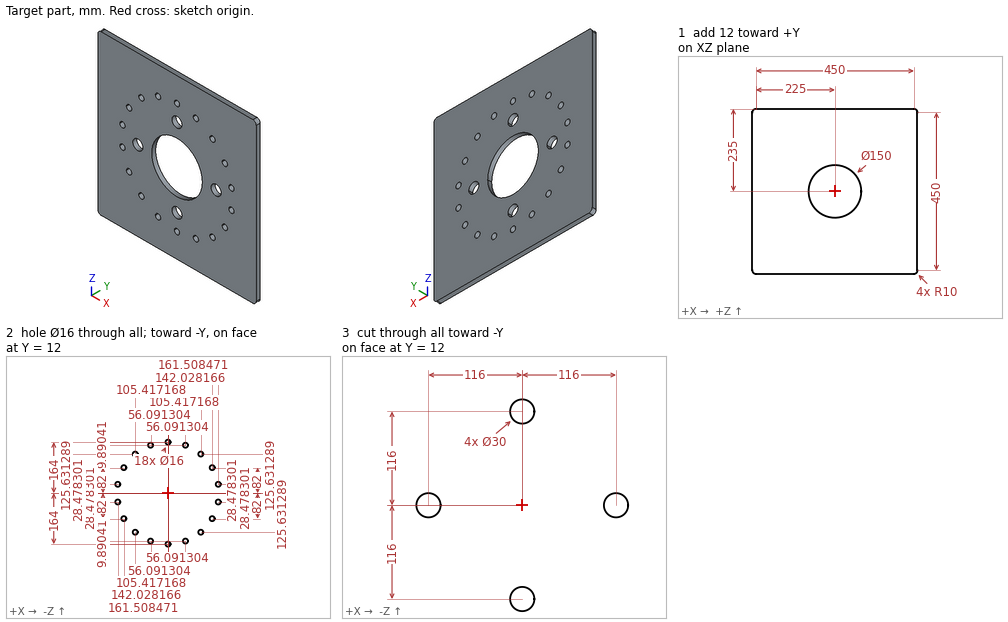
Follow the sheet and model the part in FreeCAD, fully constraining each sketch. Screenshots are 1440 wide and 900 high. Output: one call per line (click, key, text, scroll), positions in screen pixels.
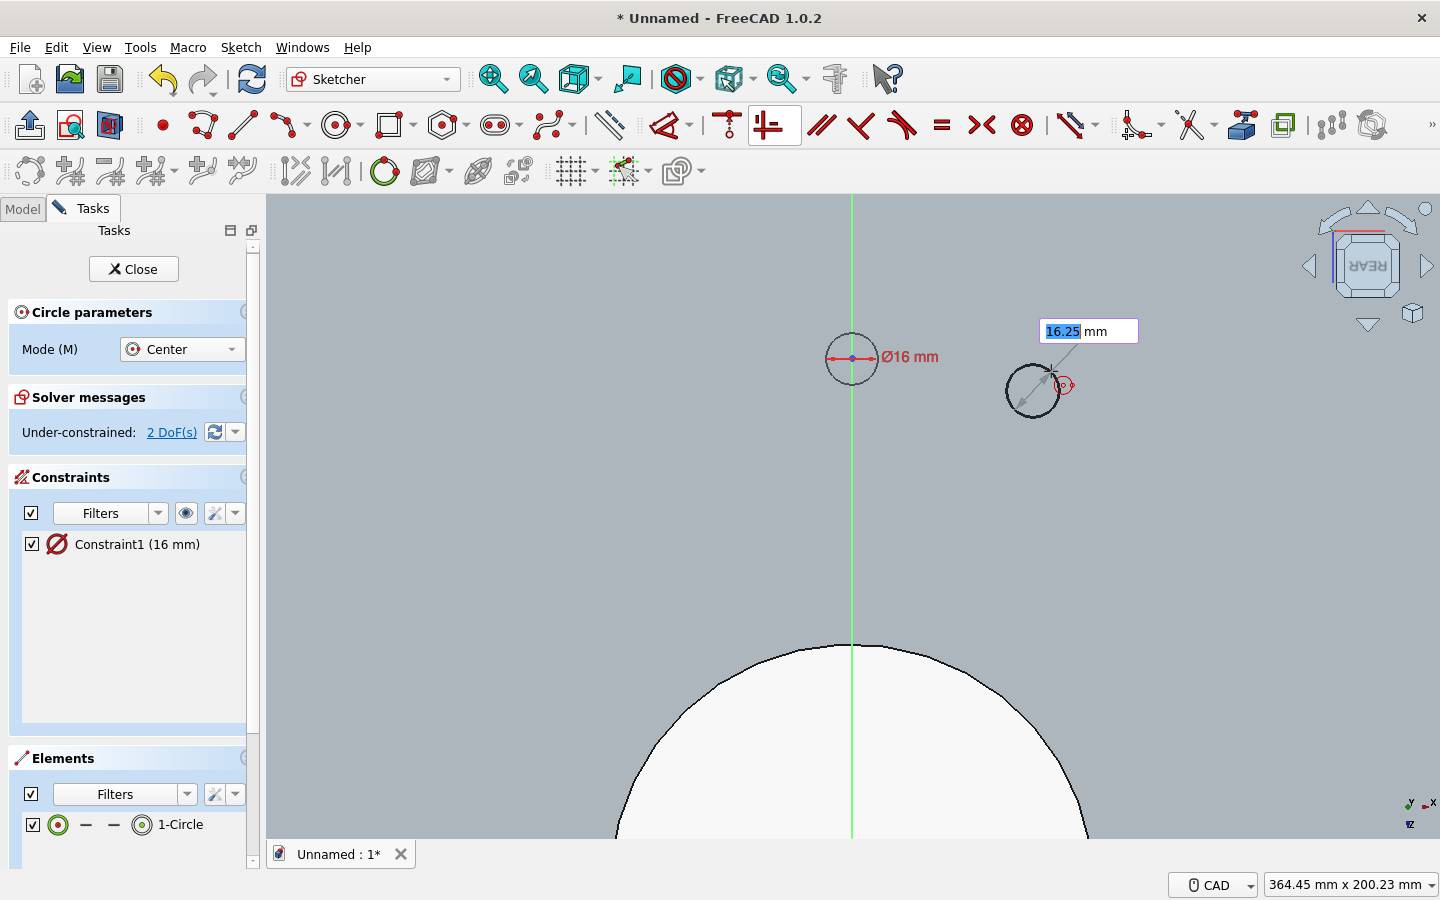
text(16)
key(Return)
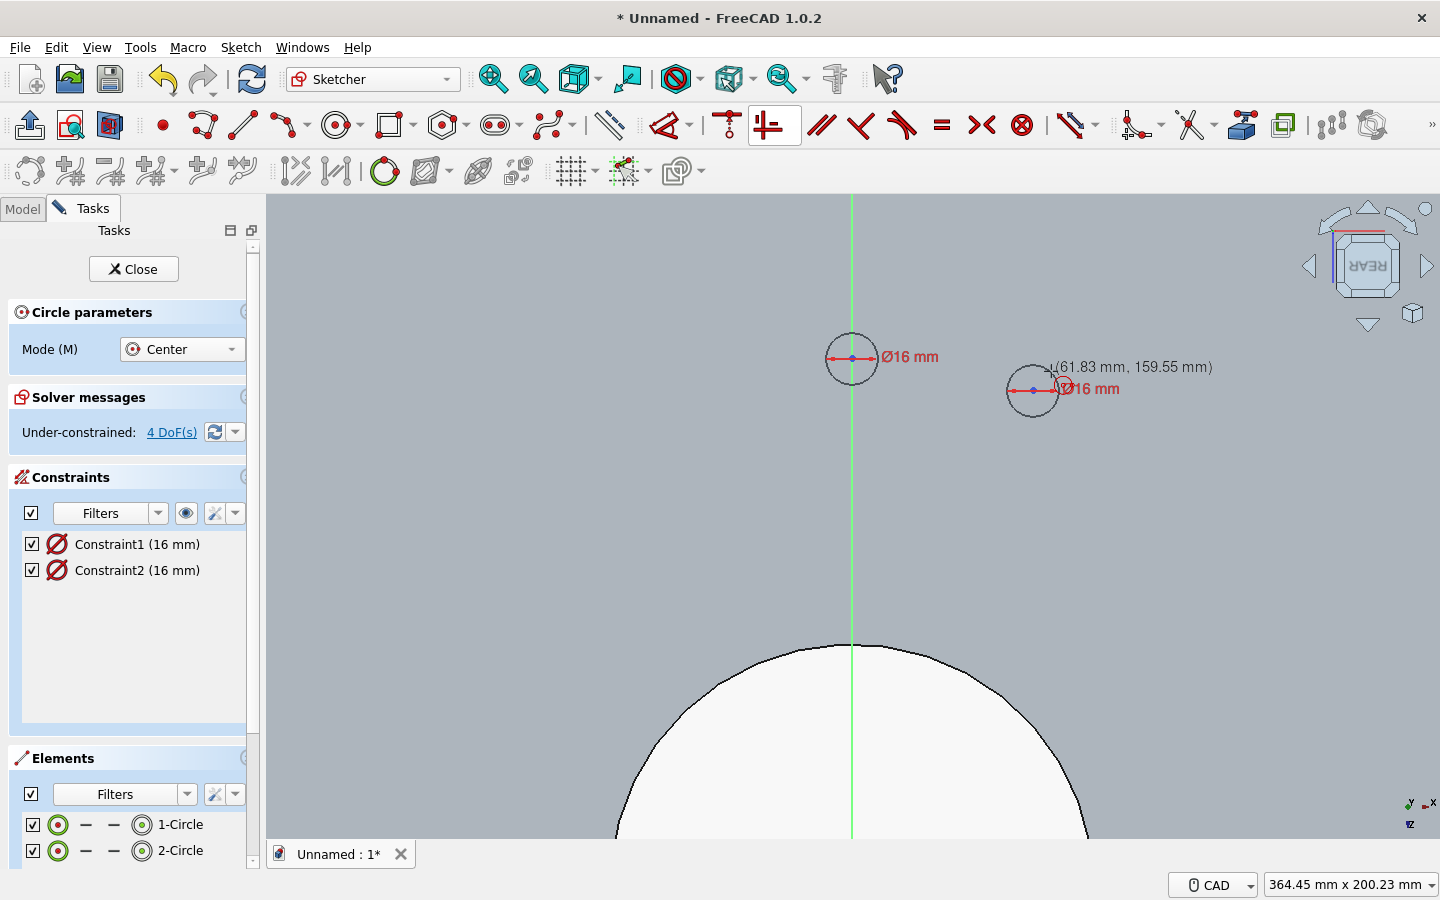
click(1191, 481)
move(1210, 463)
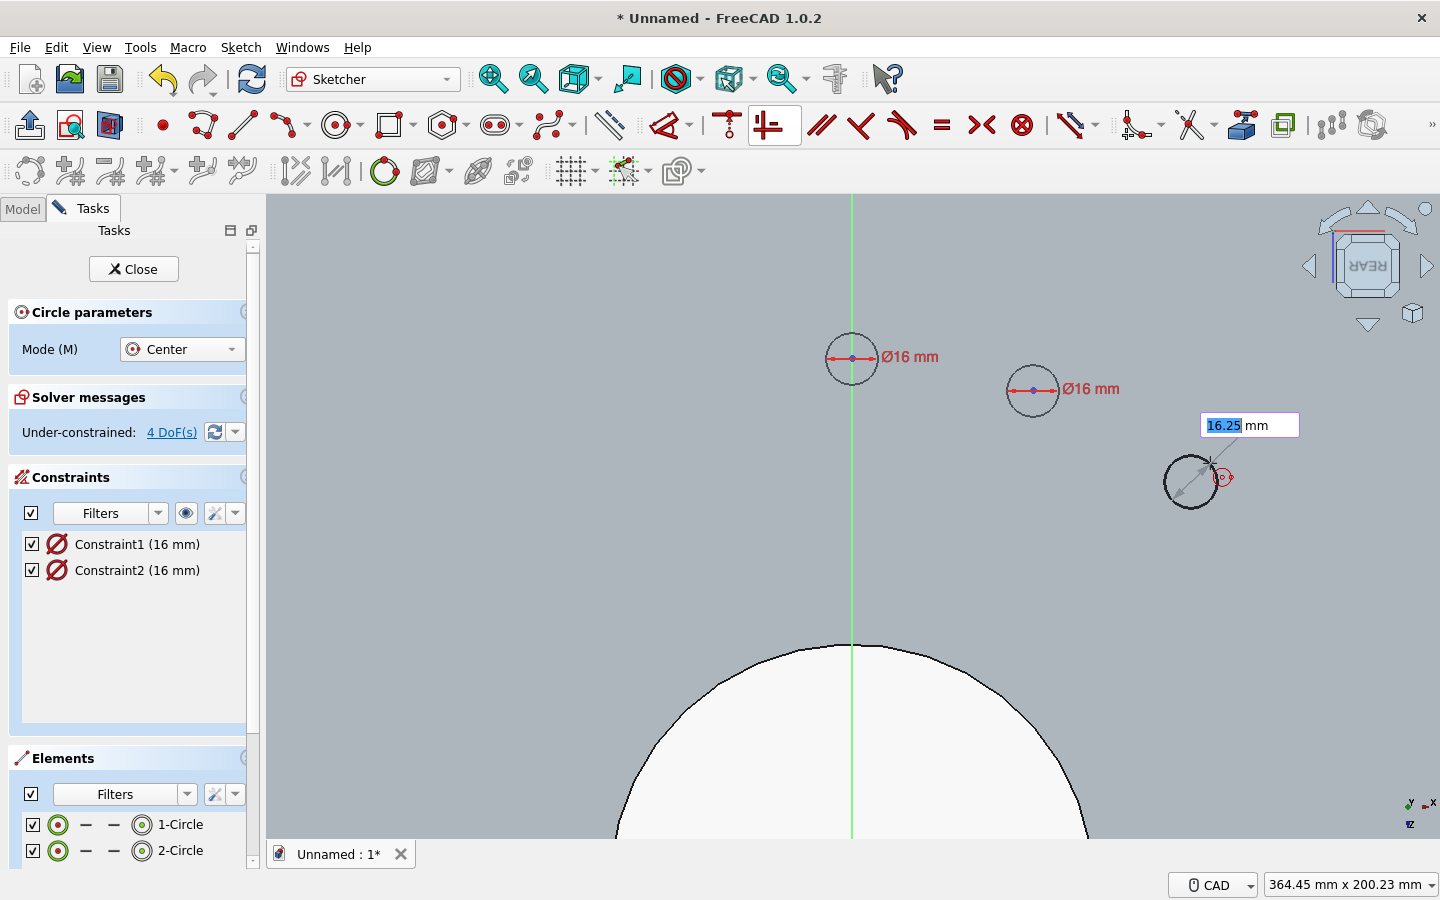
text(16)
key(Return)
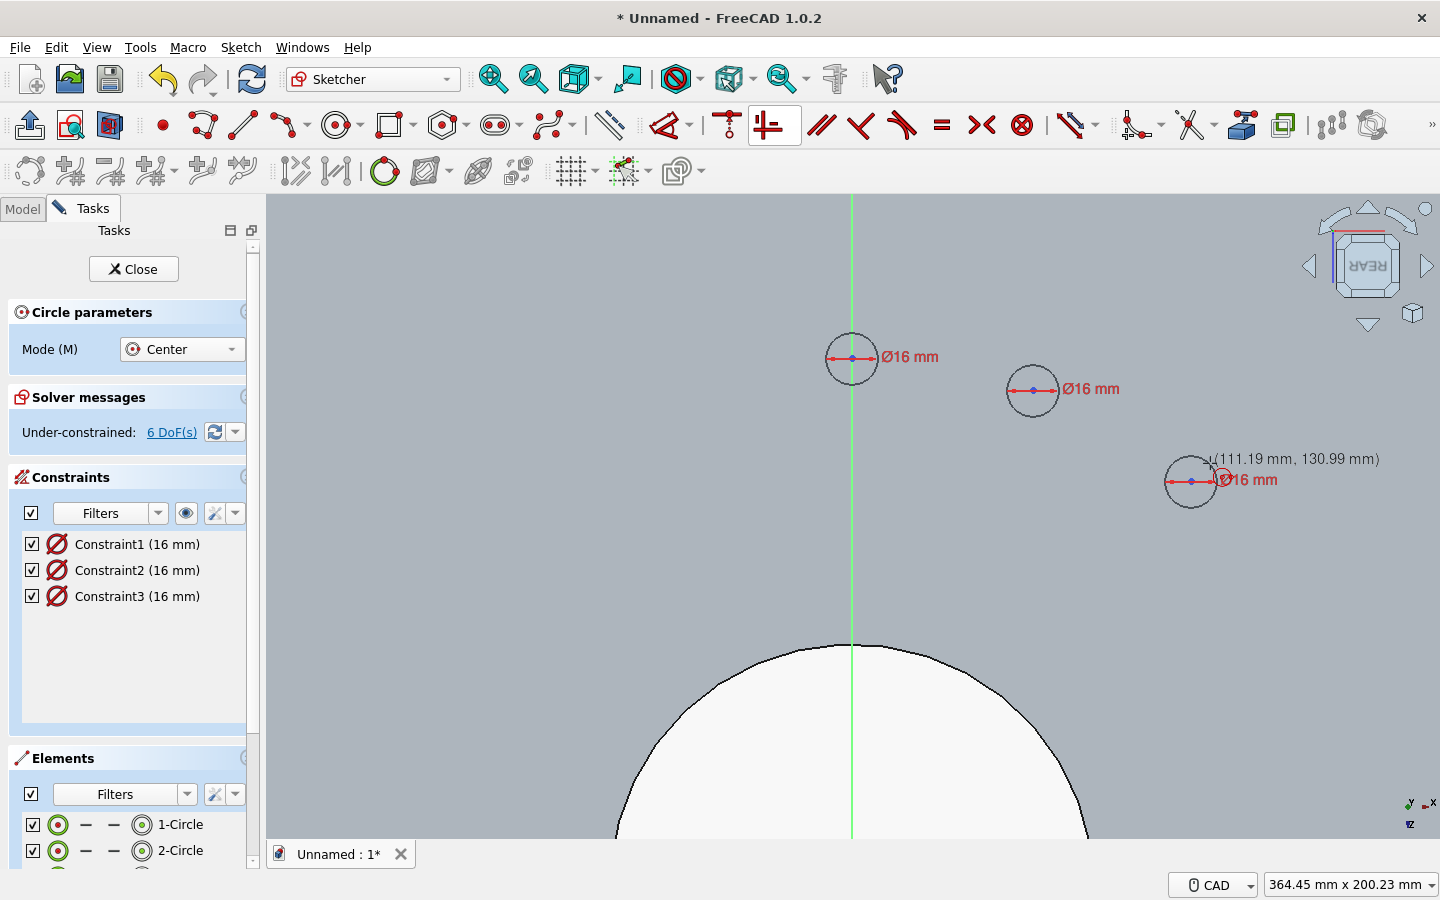
scroll(745, 301, down, 5)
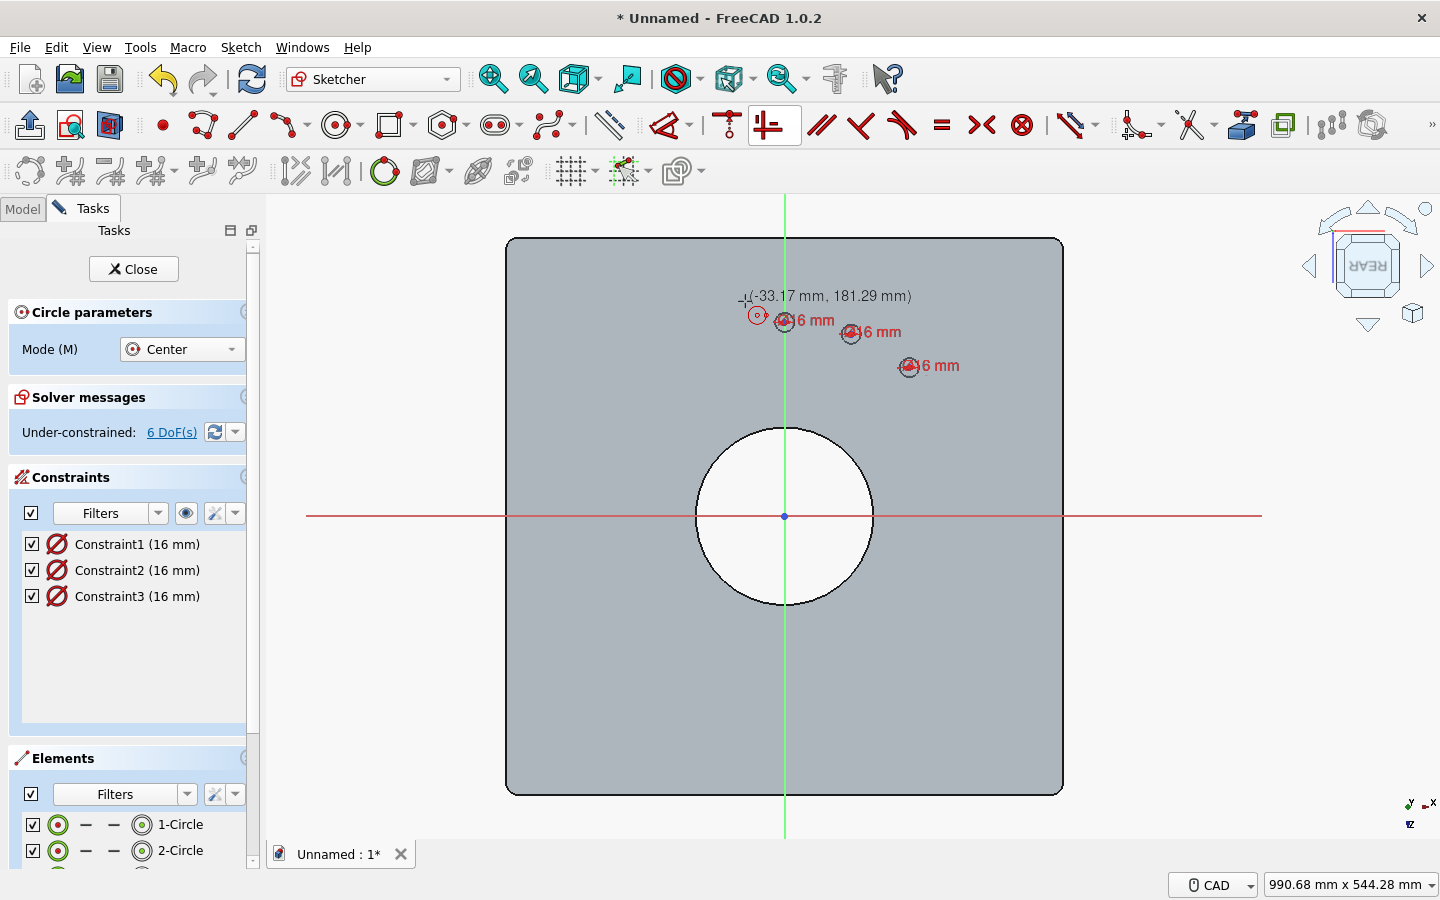
scroll(953, 419, up, 5)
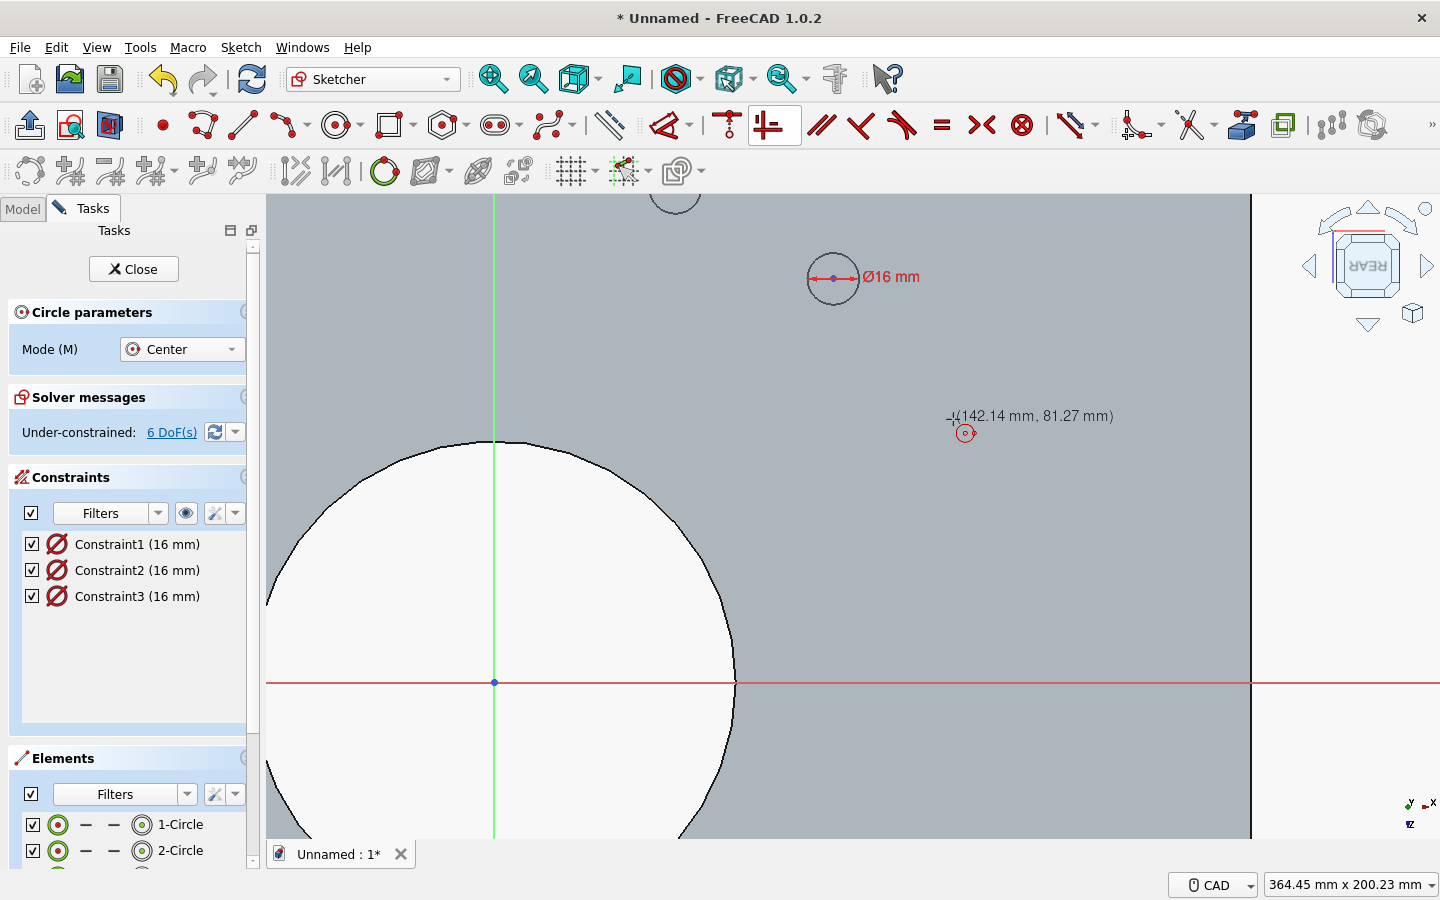
click(952, 419)
move(970, 401)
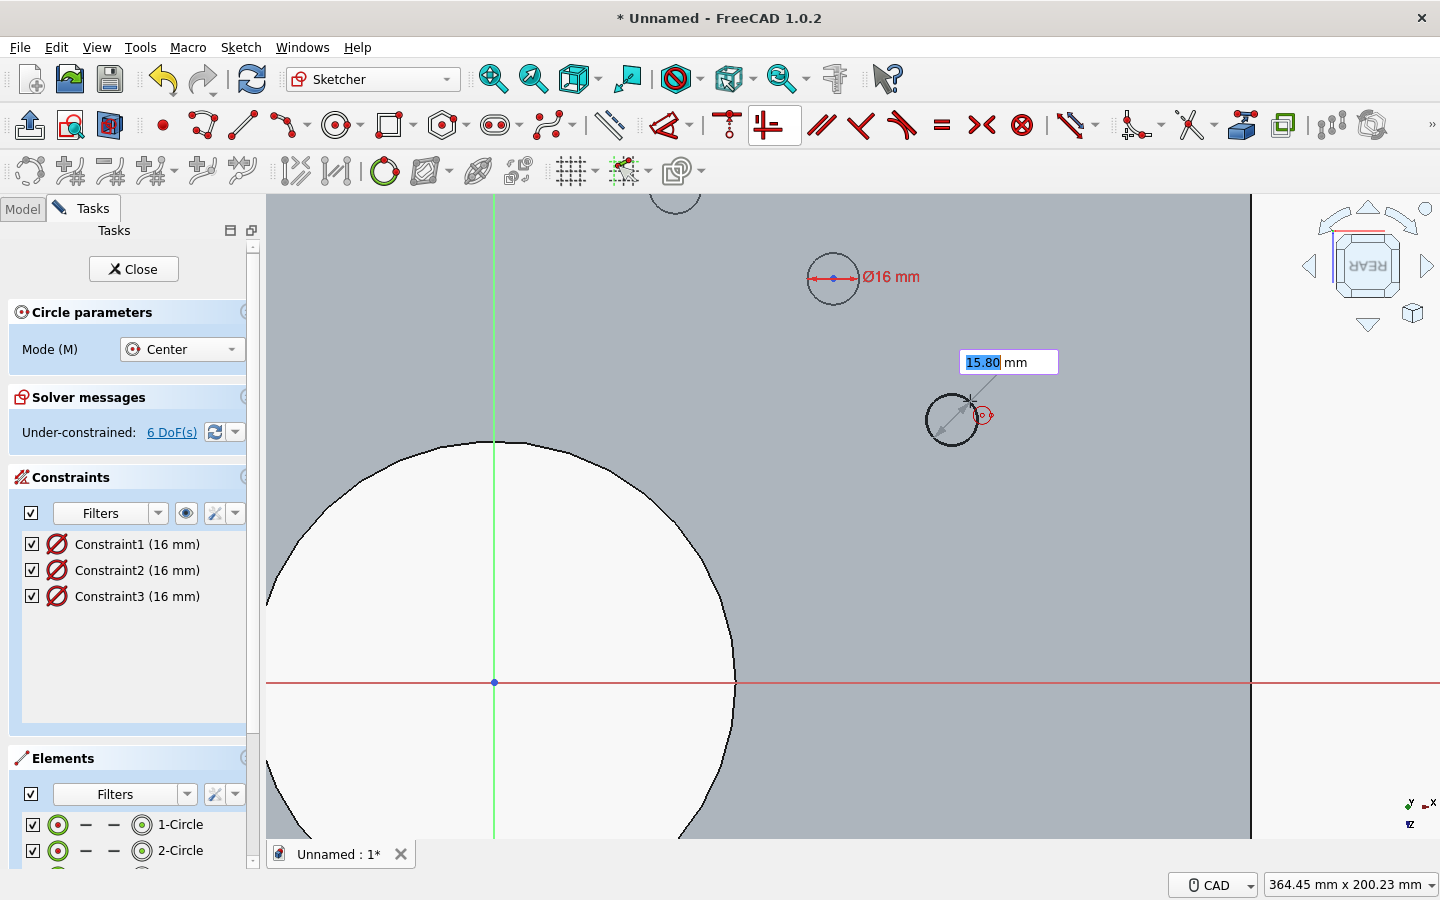
text(16)
key(Return)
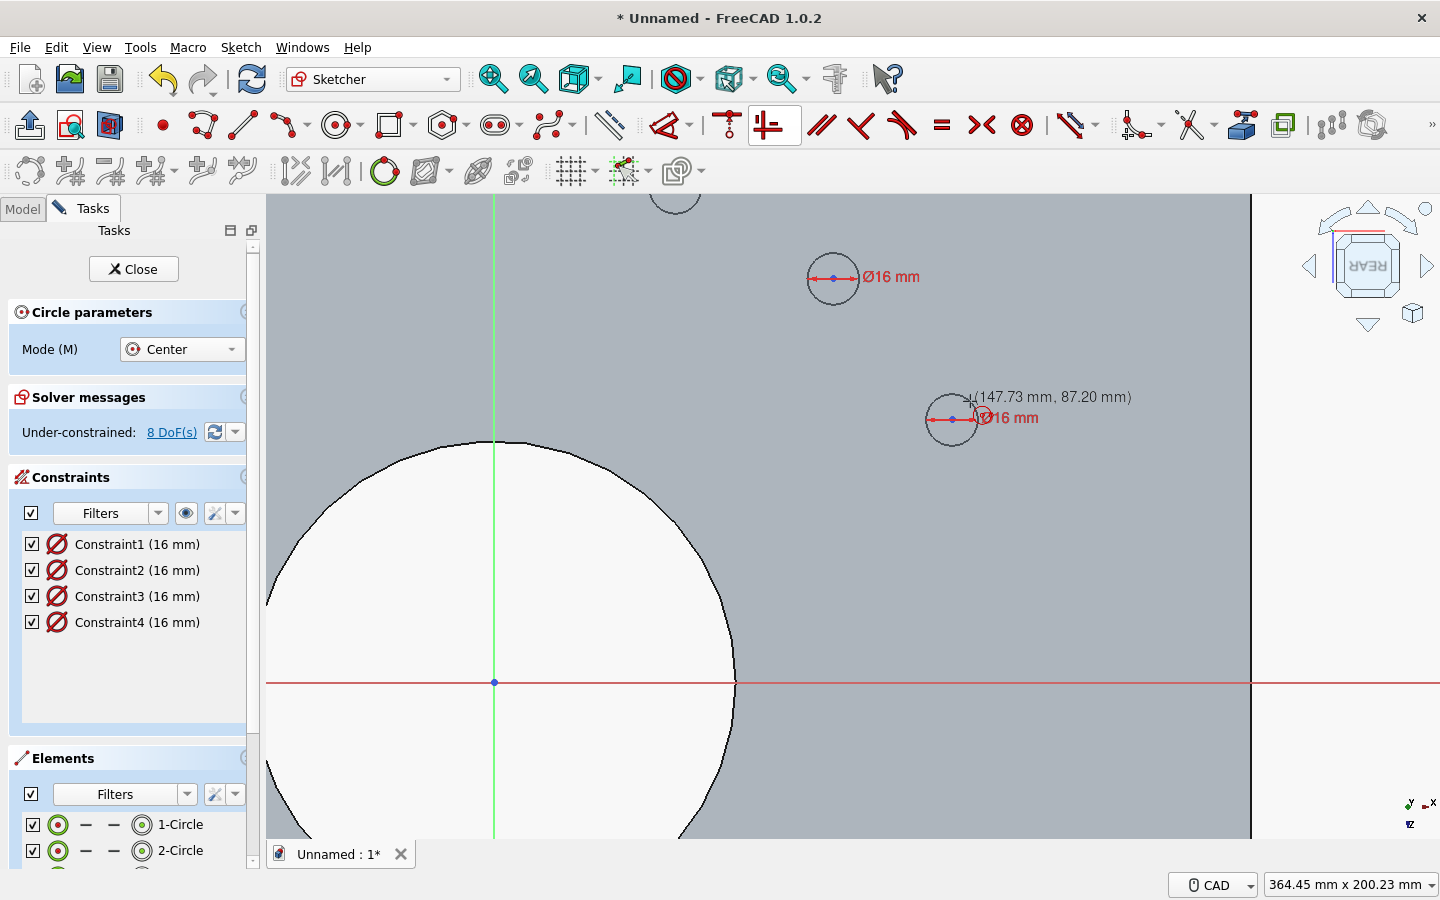
click(1014, 591)
move(1033, 573)